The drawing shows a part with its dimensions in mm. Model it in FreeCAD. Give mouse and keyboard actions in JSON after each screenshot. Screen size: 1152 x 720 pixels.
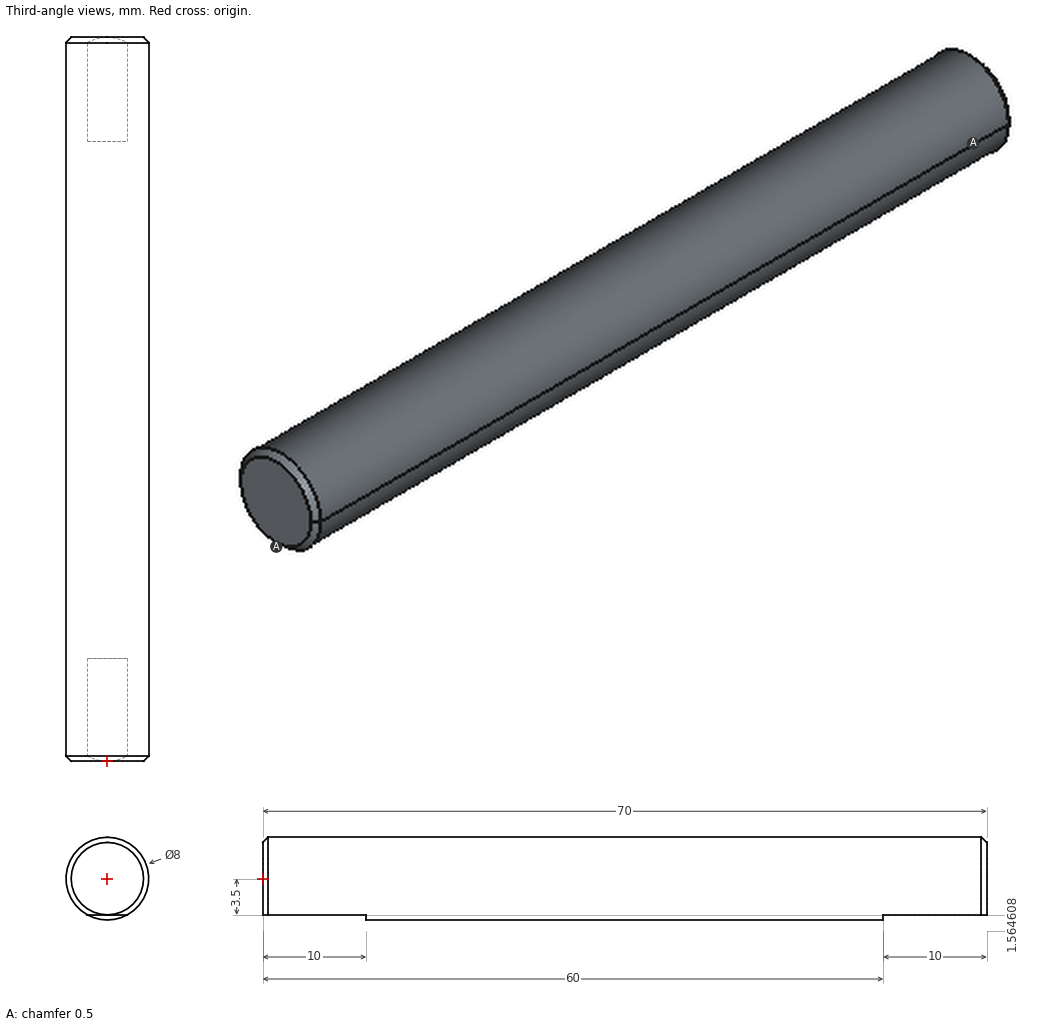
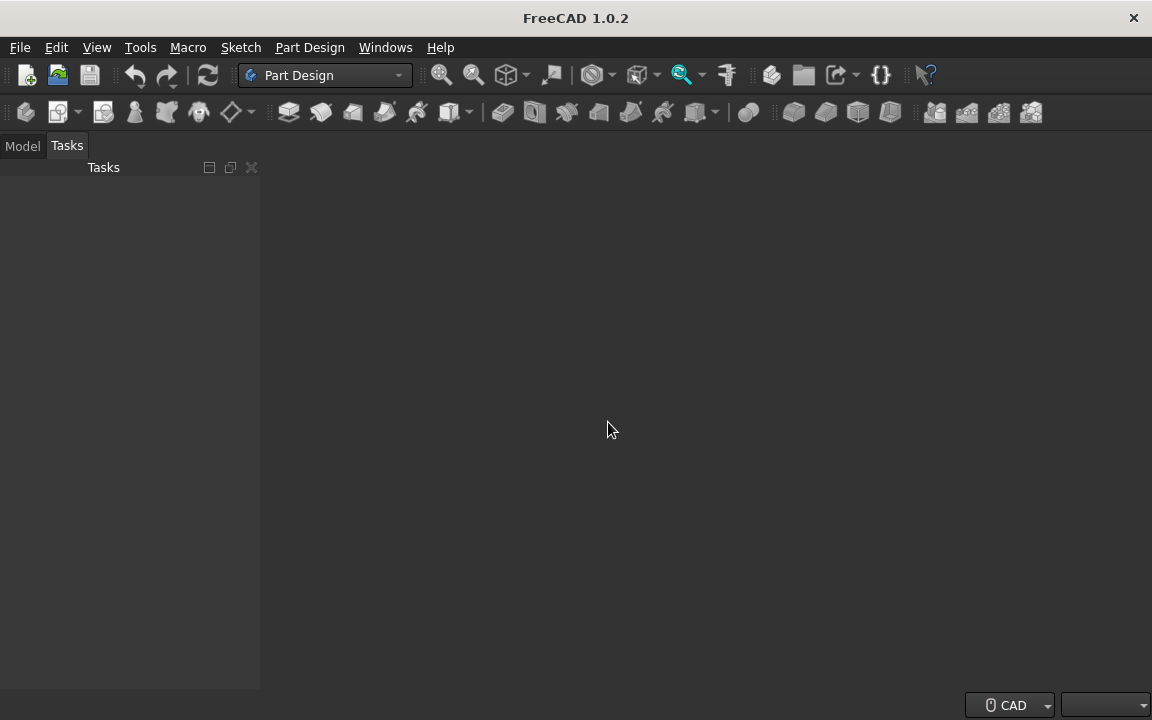
{"action": "left_click", "coordinate": [26, 76]}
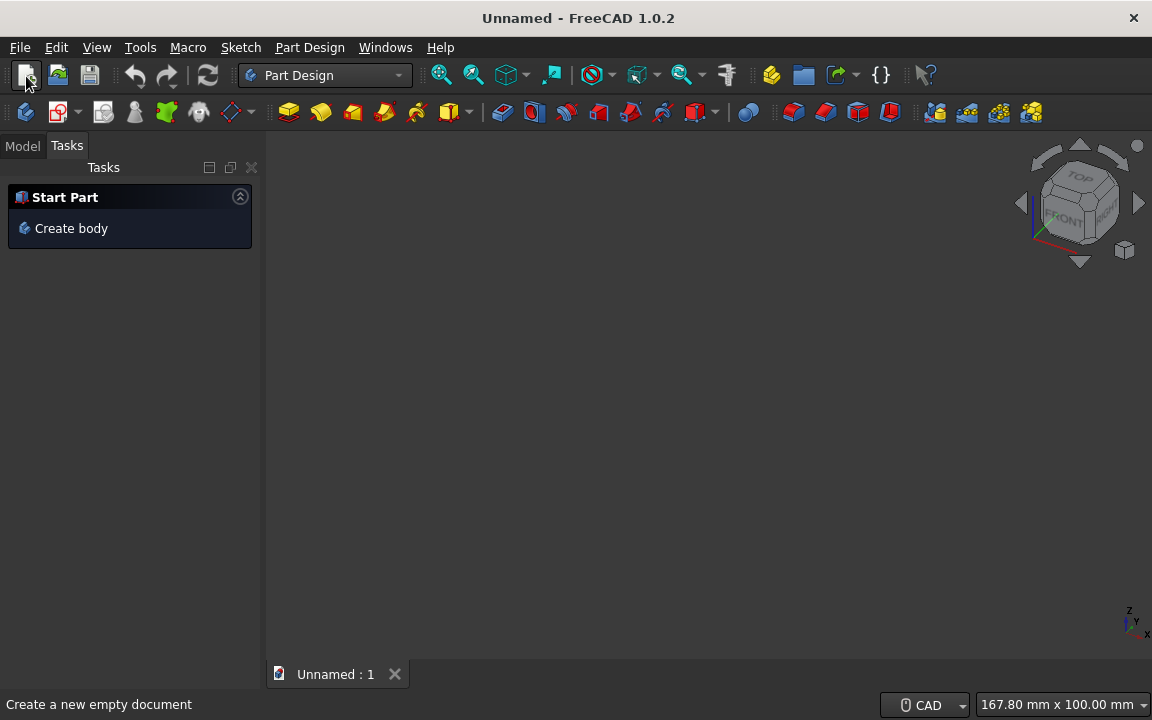
{"action": "left_click", "coordinate": [58, 112]}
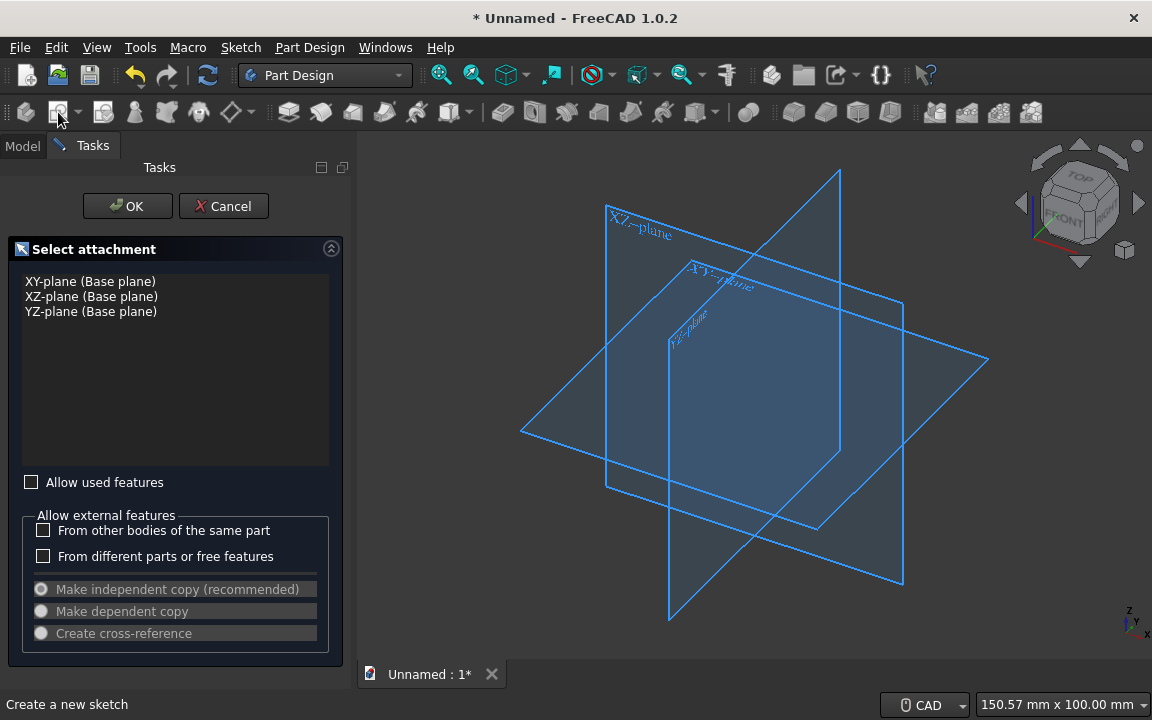
{"action": "left_click", "coordinate": [82, 296]}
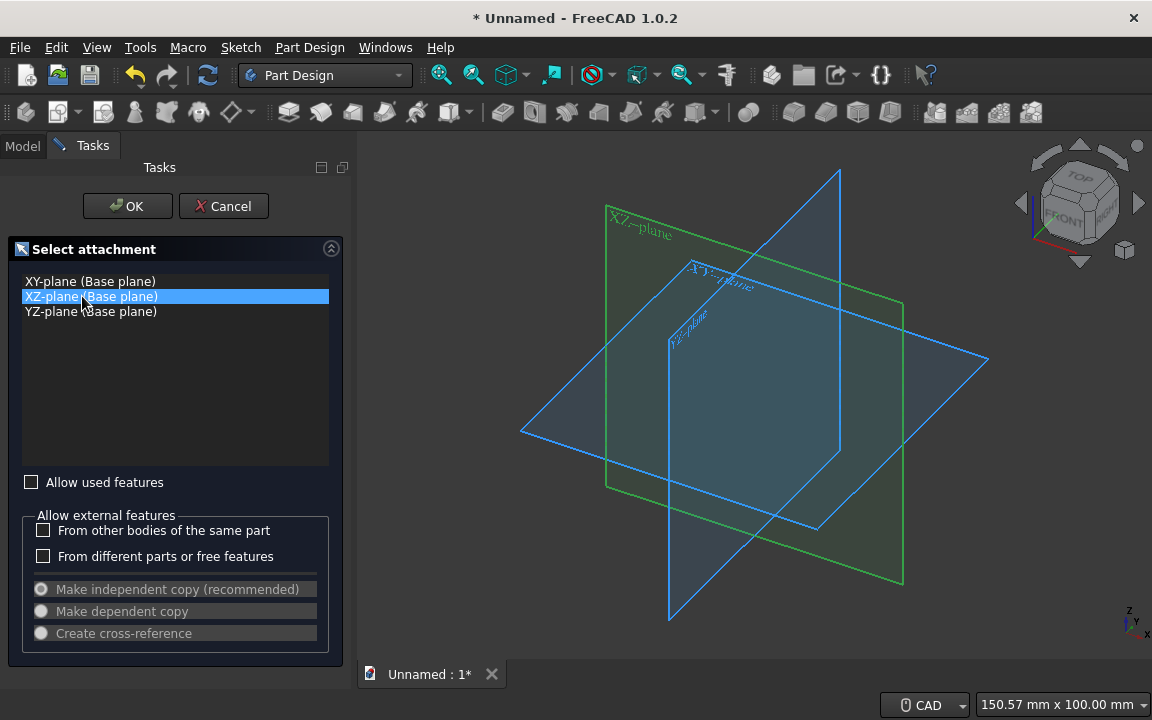
{"action": "left_click", "coordinate": [128, 206]}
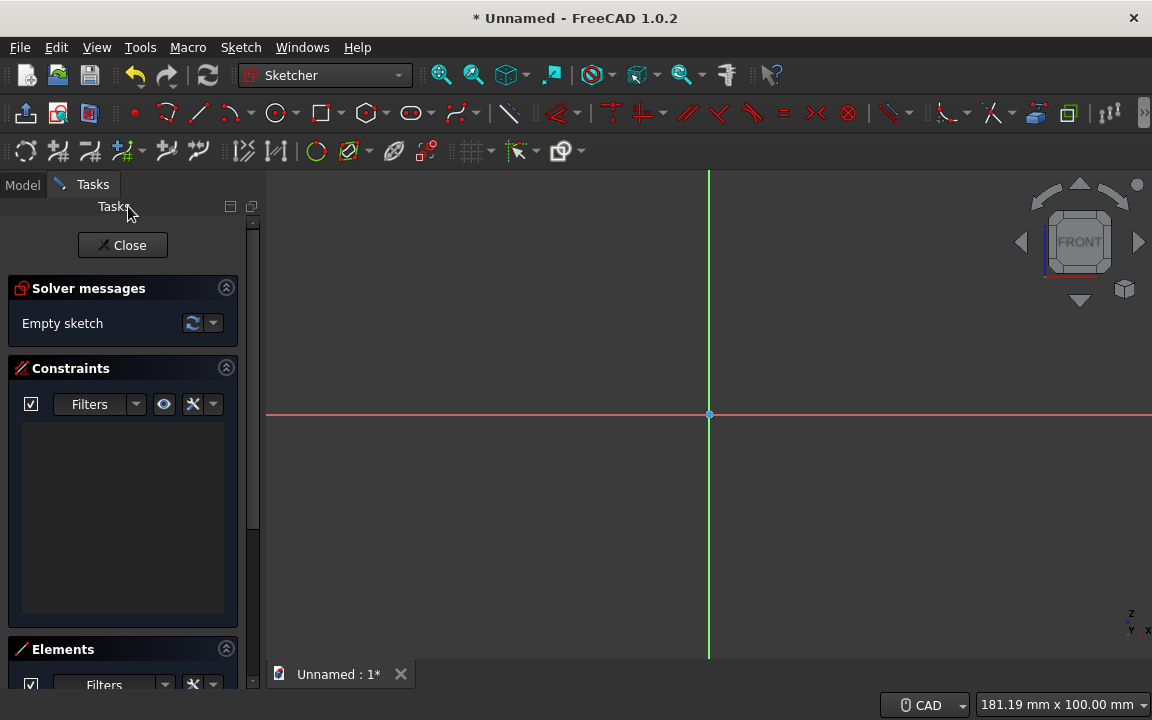
{"action": "scroll", "coordinate": [720, 414], "scroll_direction": "up", "scroll_amount": 10}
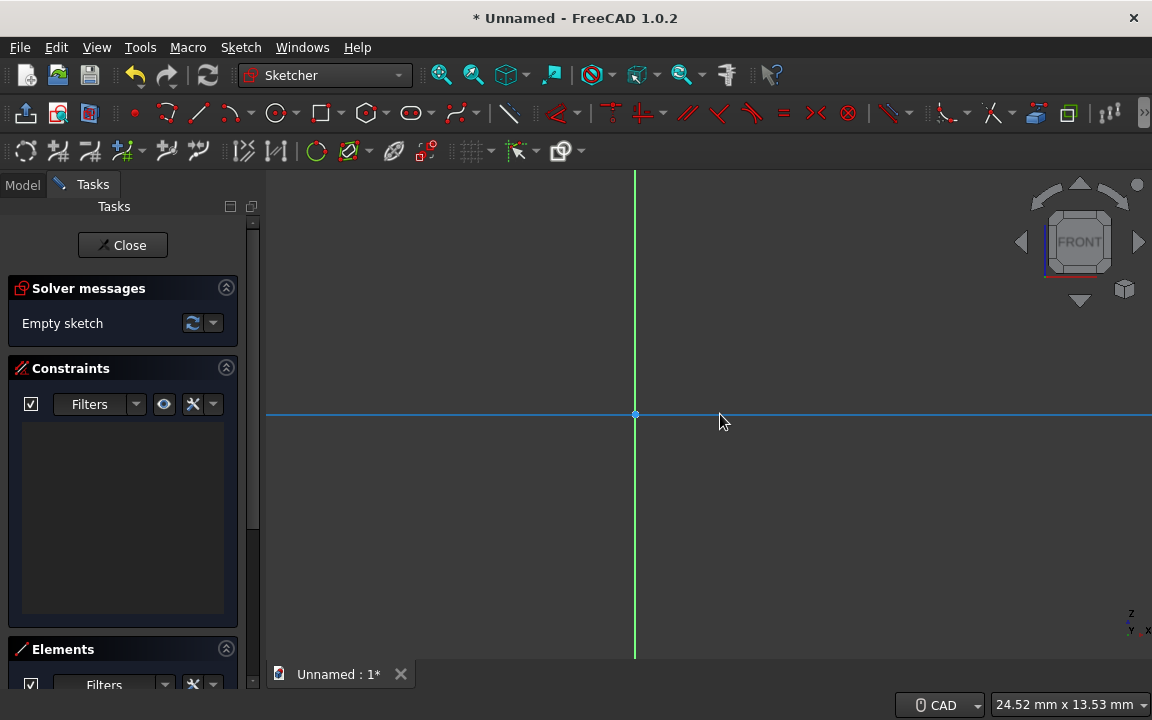
{"action": "left_click", "coordinate": [276, 114]}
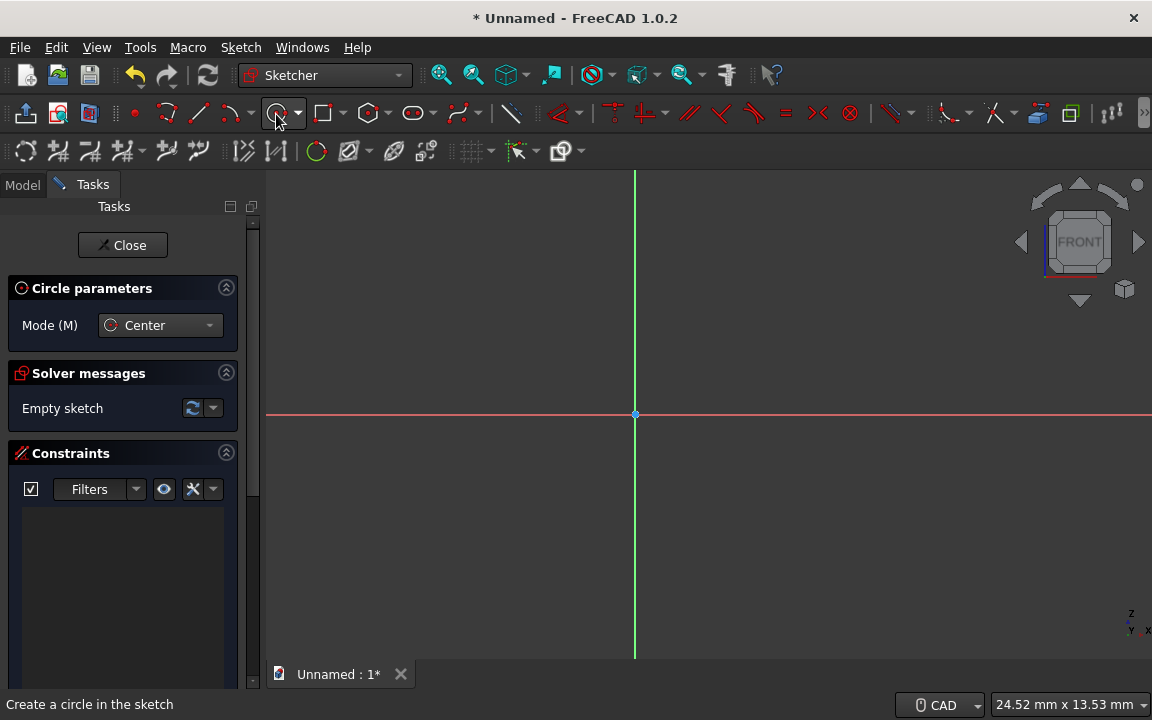
{"action": "left_click", "coordinate": [635, 414]}
{"action": "mouse_move", "coordinate": [738, 312]}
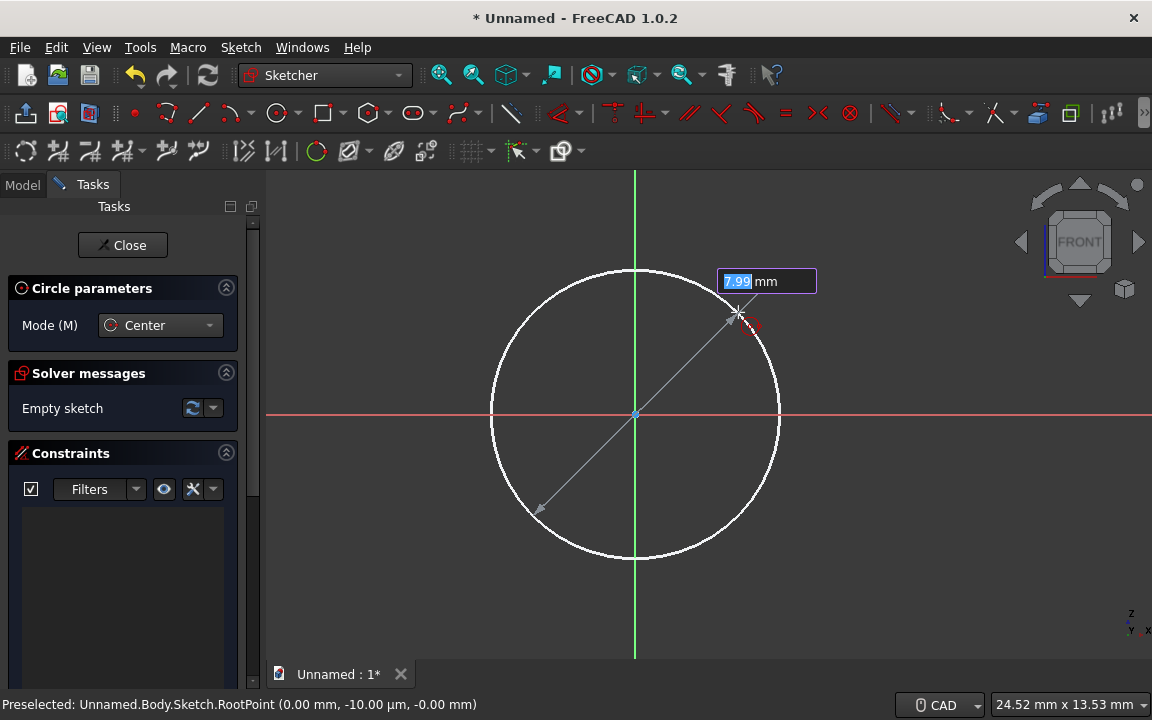
{"action": "type", "text": "8"}
{"action": "key", "text": "Return"}
{"action": "key", "text": "Escape"}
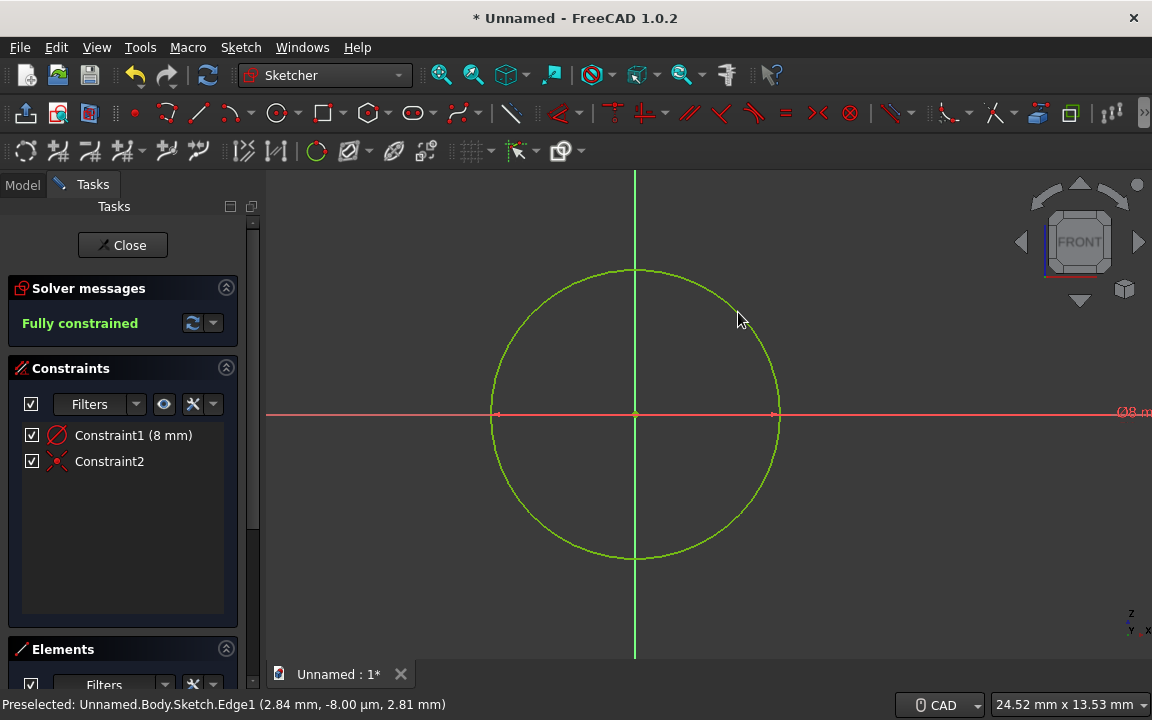
{"action": "left_click", "coordinate": [123, 245]}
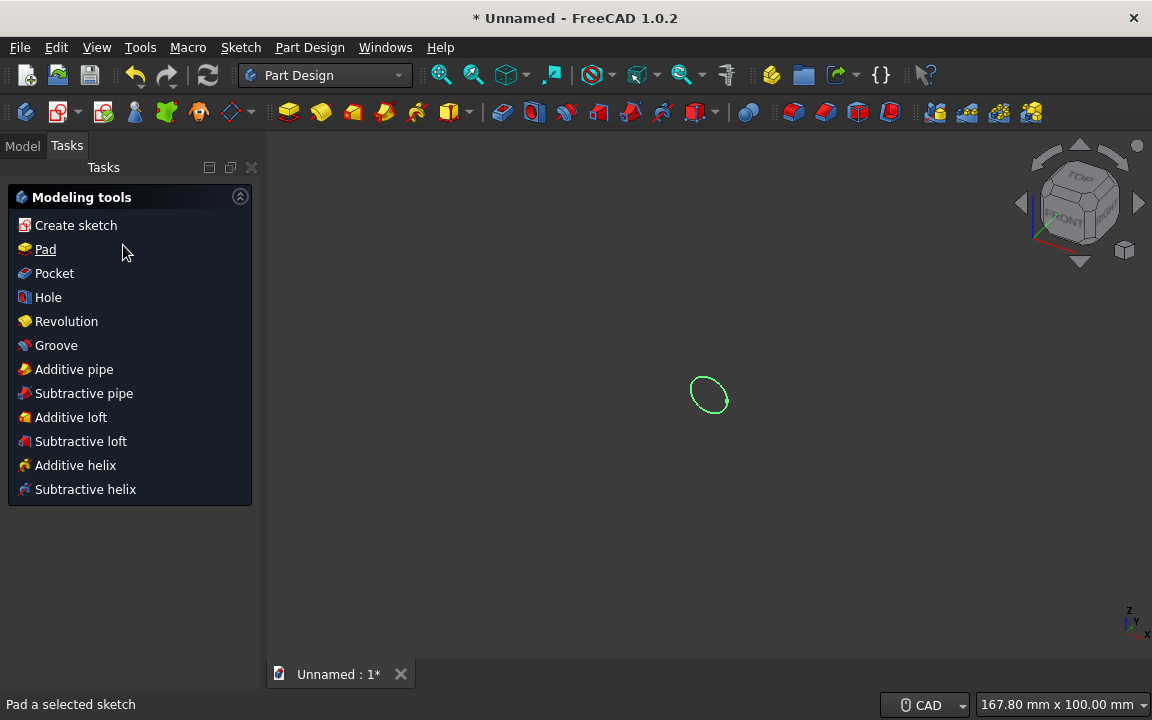
{"action": "left_click", "coordinate": [290, 112]}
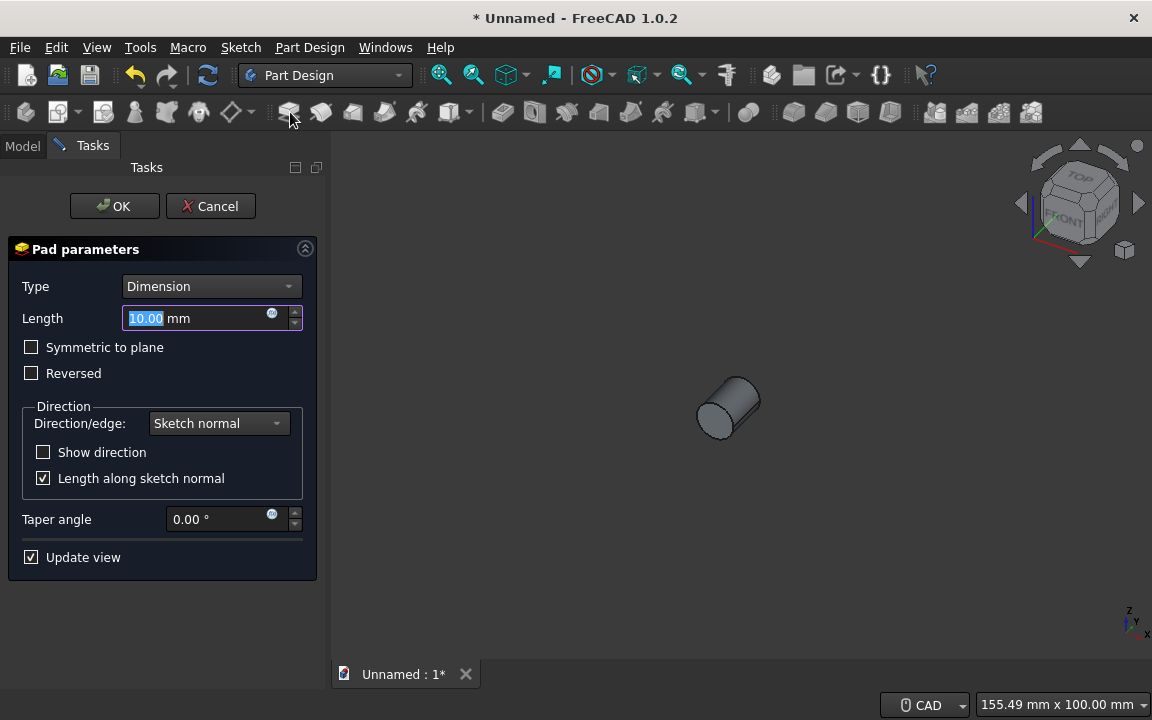
{"action": "type", "text": "70"}
{"action": "key", "text": "Tab"}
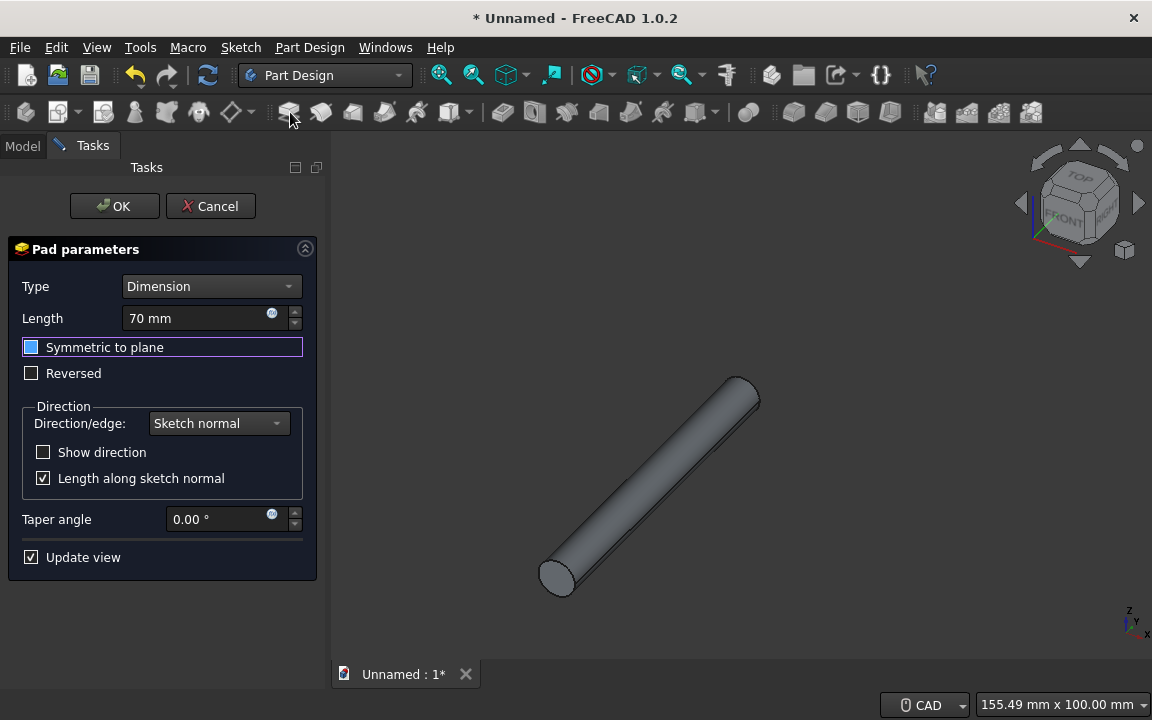
{"action": "left_click", "coordinate": [30, 373]}